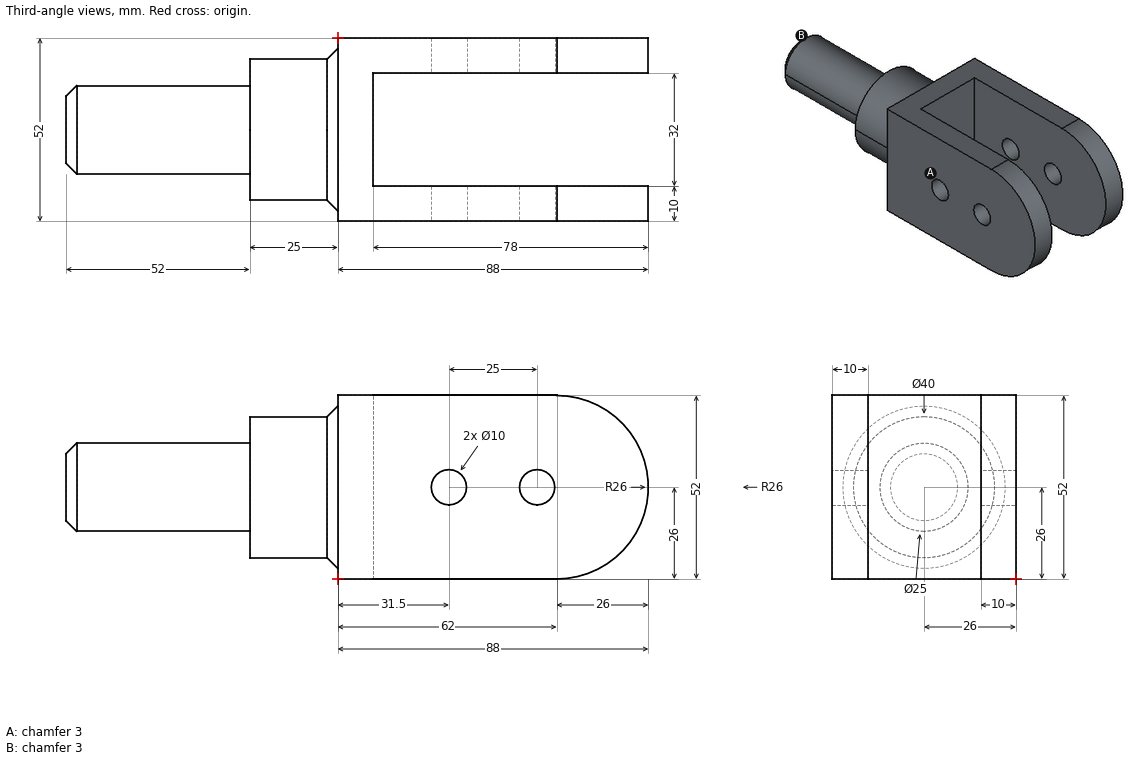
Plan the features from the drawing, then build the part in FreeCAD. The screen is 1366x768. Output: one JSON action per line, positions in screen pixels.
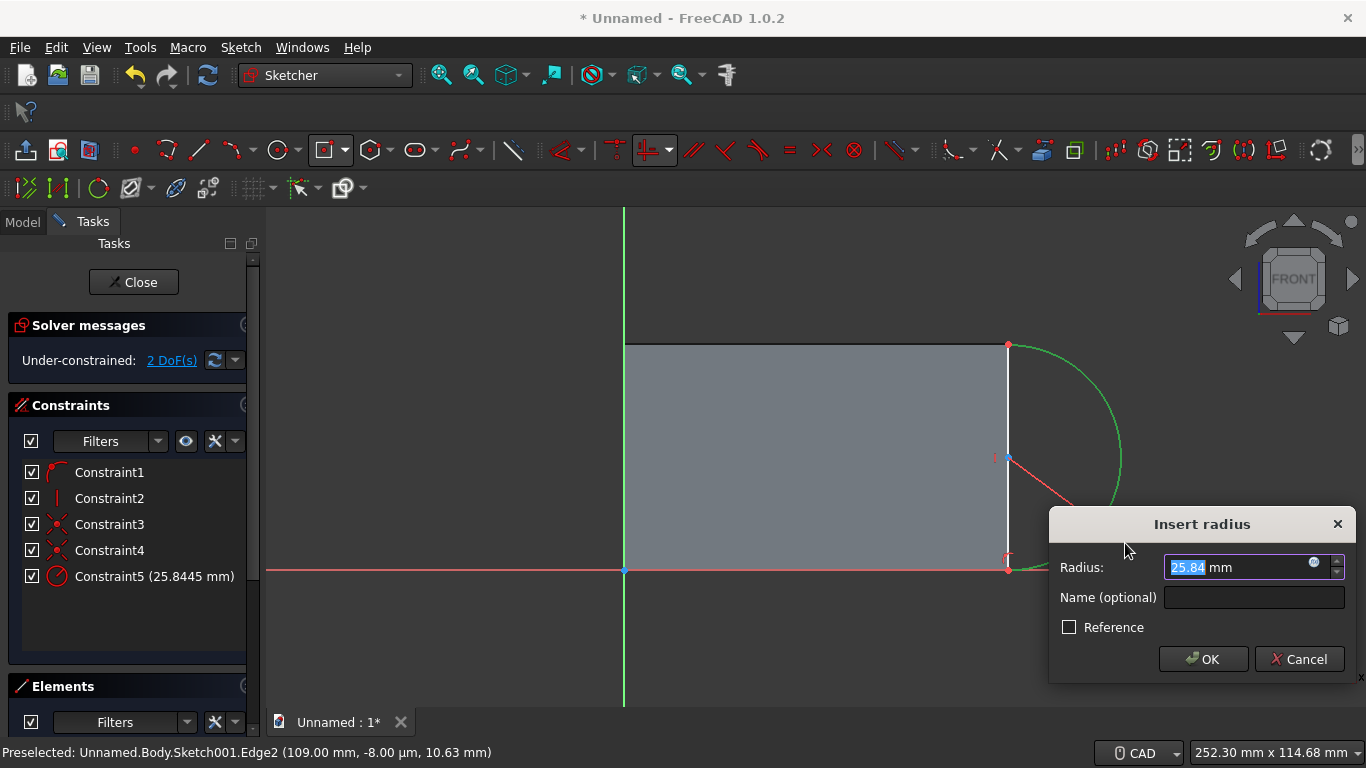
{"action": "type", "text": "26"}
{"action": "key", "text": "Return"}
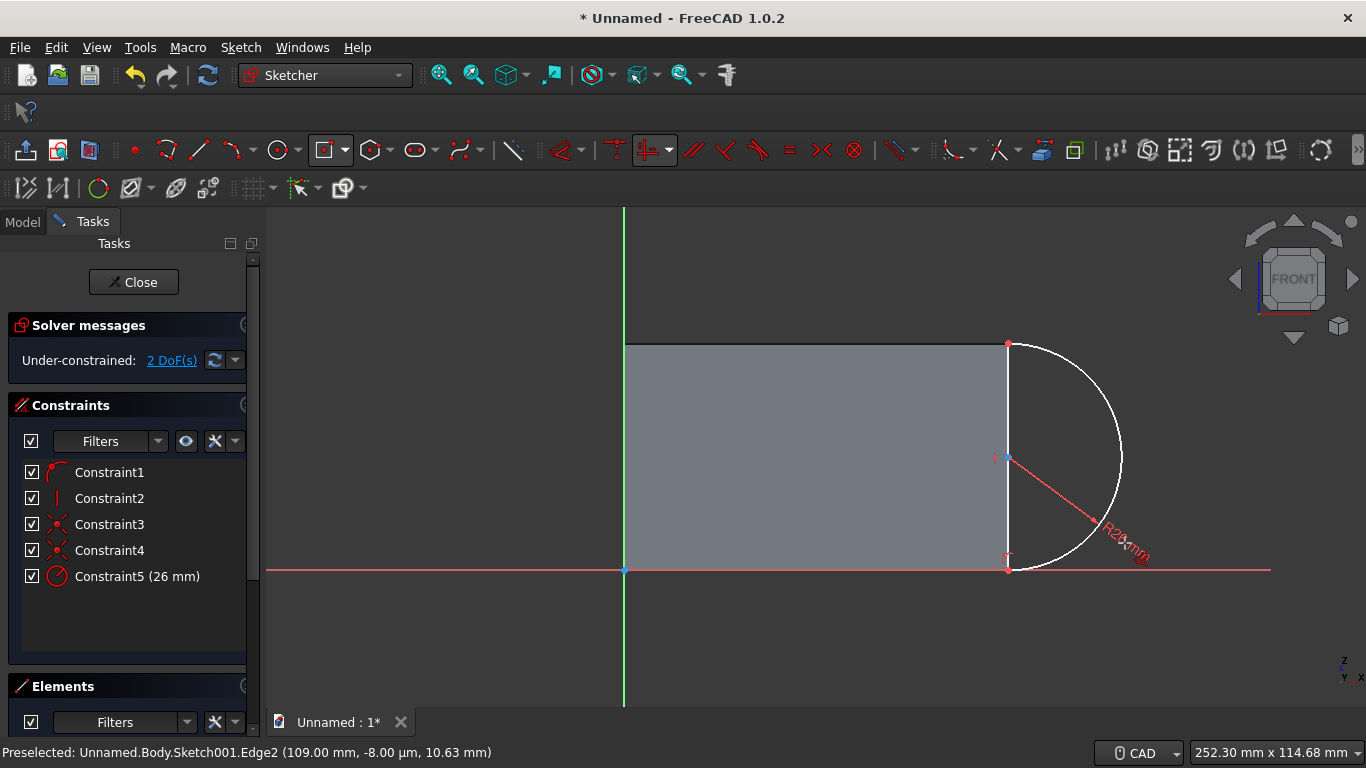
{"action": "left_click", "coordinate": [1008, 570]}
{"action": "left_click", "coordinate": [816, 604]}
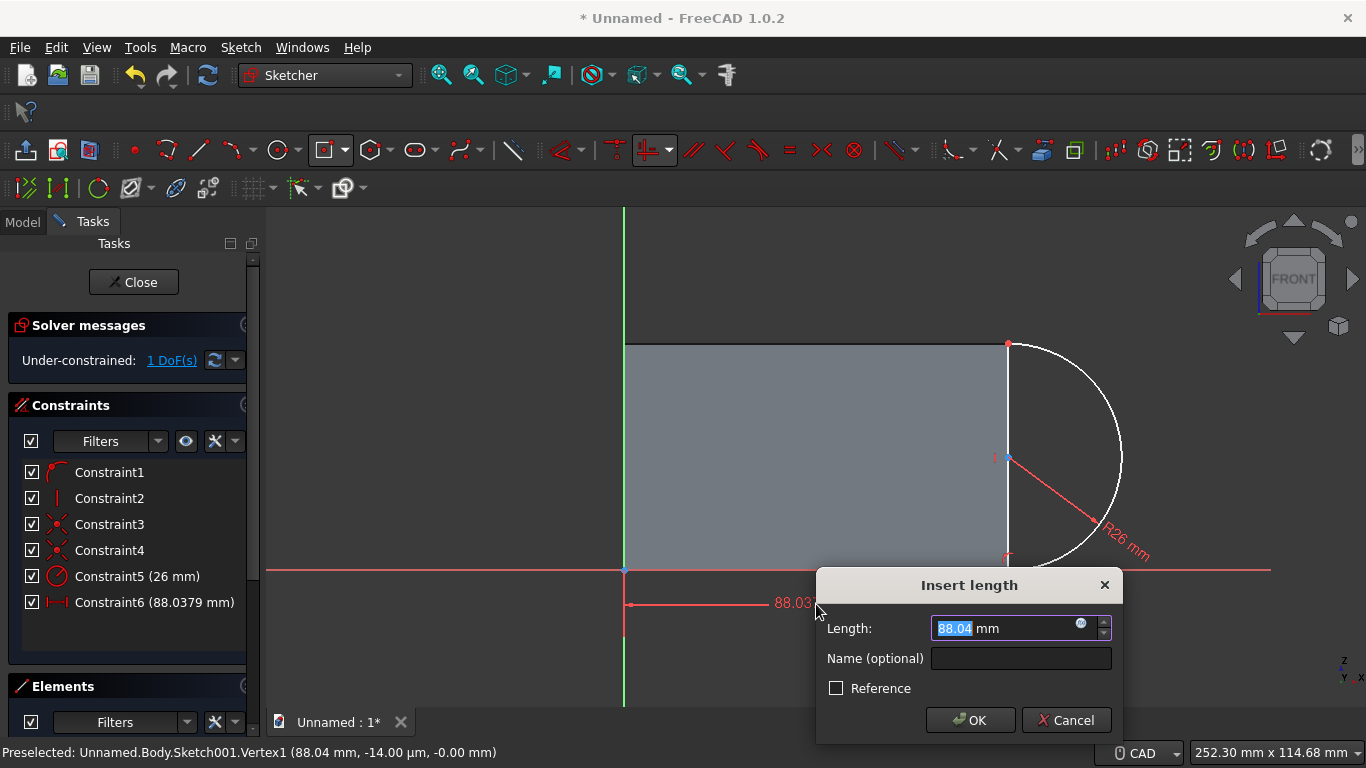
{"action": "type", "text": "88"}
{"action": "key", "text": "Return"}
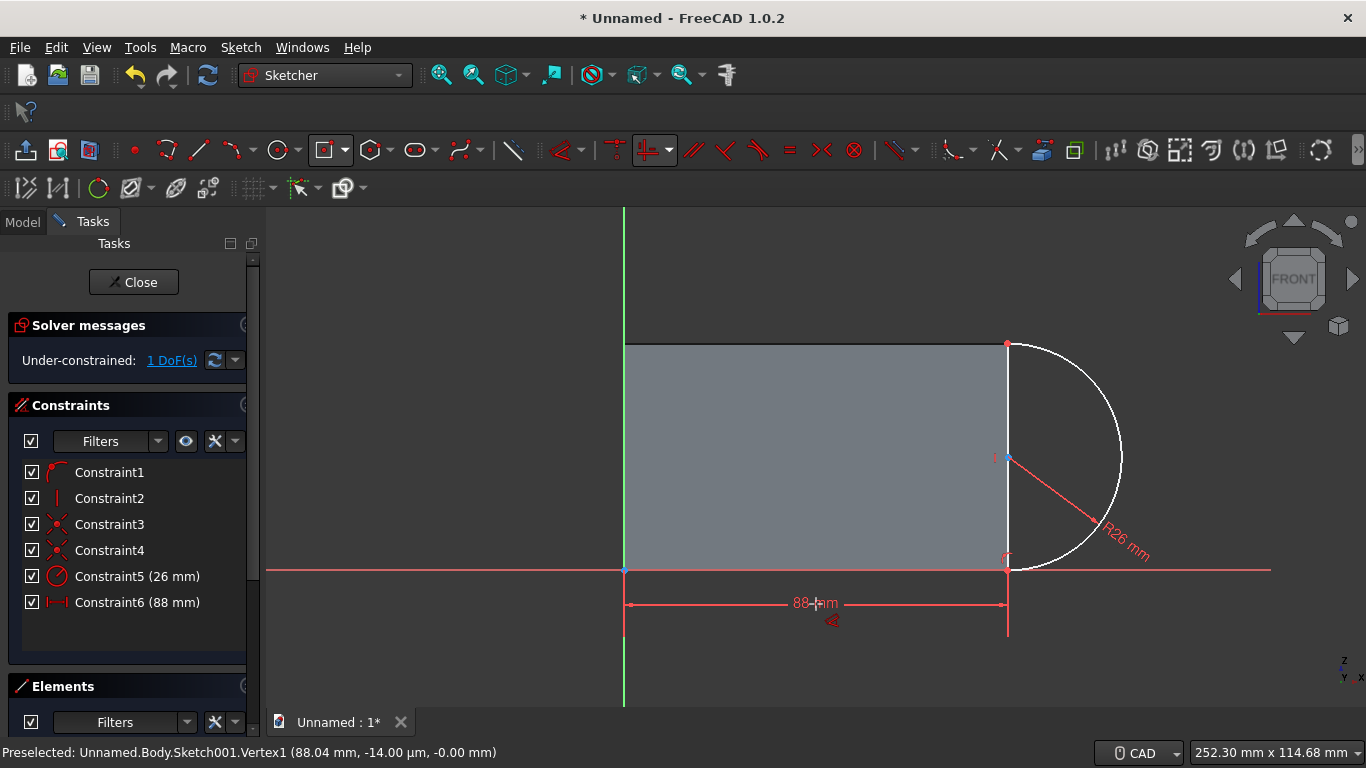
{"action": "left_click", "coordinate": [1008, 457]}
{"action": "left_click", "coordinate": [728, 604]}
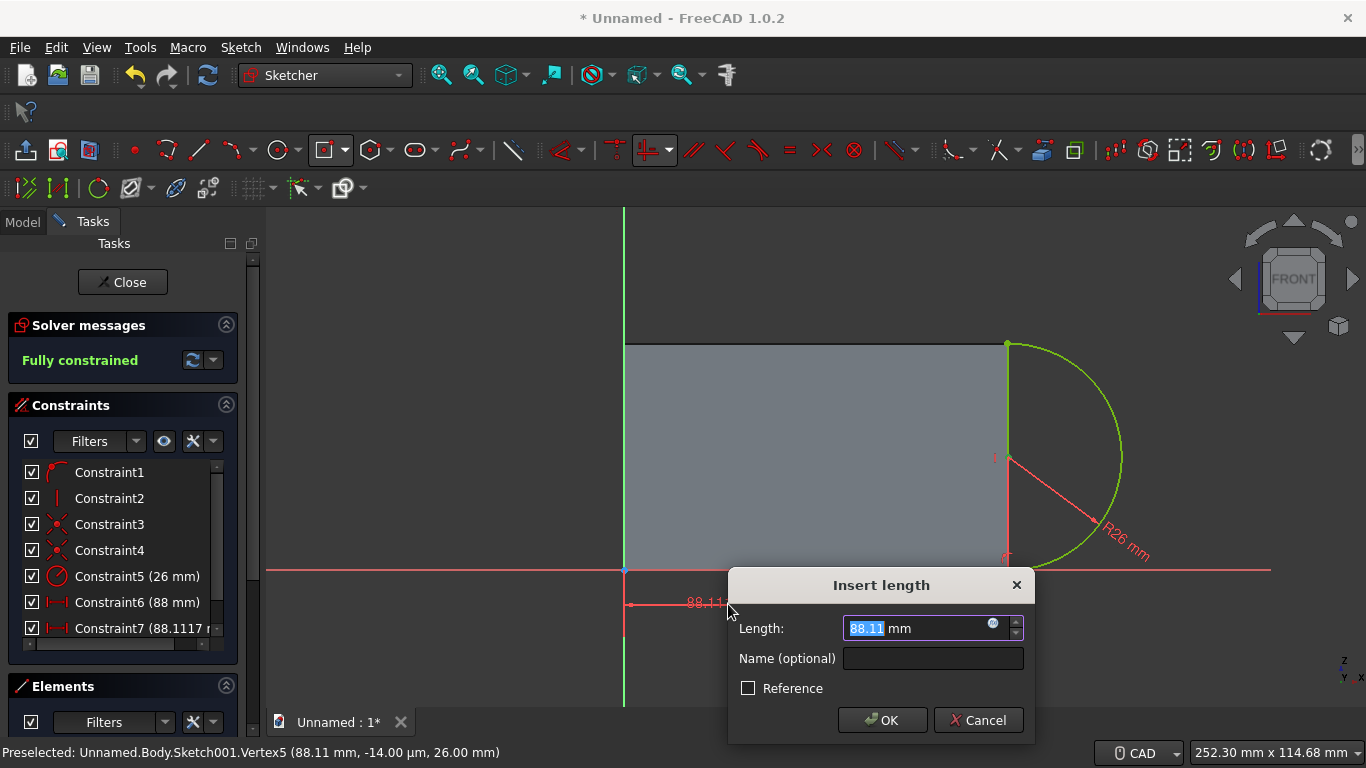
{"action": "type", "text": "88"}
{"action": "key", "text": "Return"}
{"action": "key", "text": "Escape"}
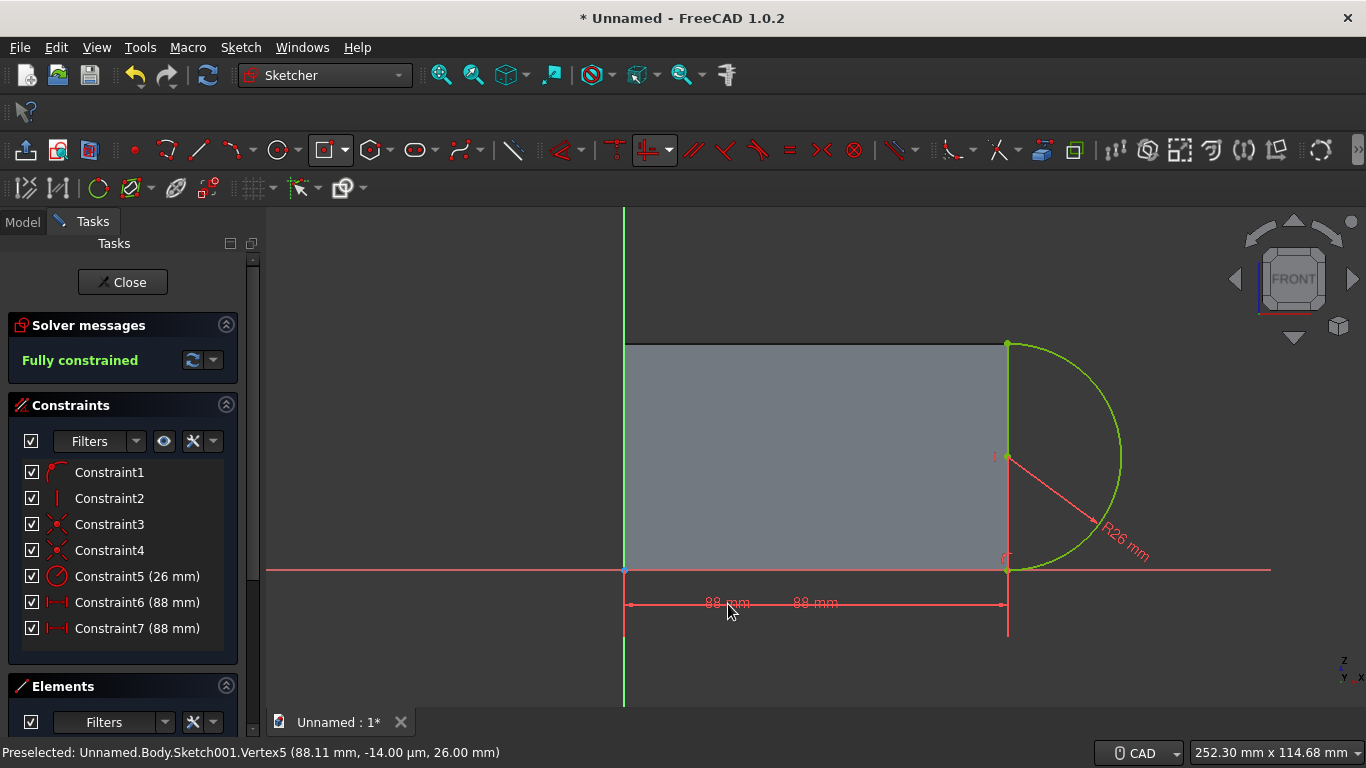
{"action": "left_click", "coordinate": [123, 282]}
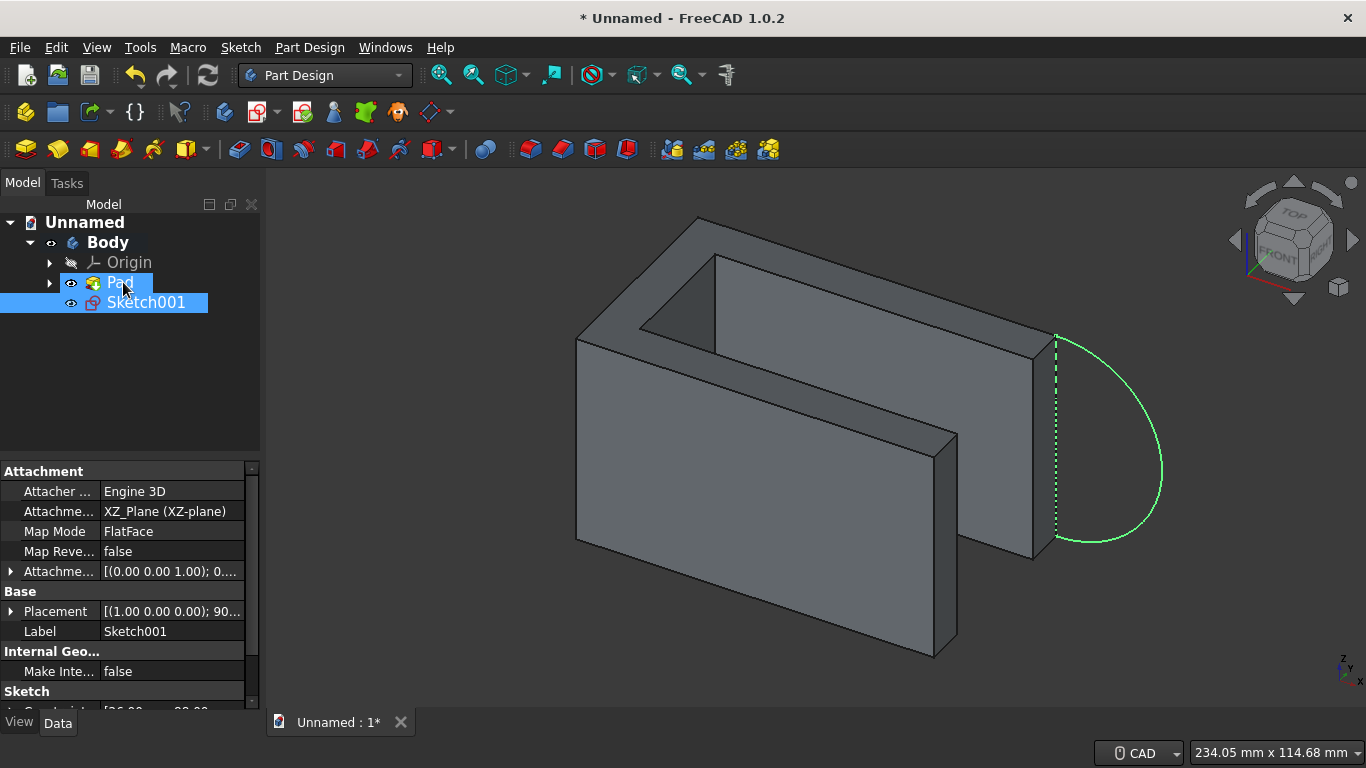
{"action": "left_click", "coordinate": [26, 150]}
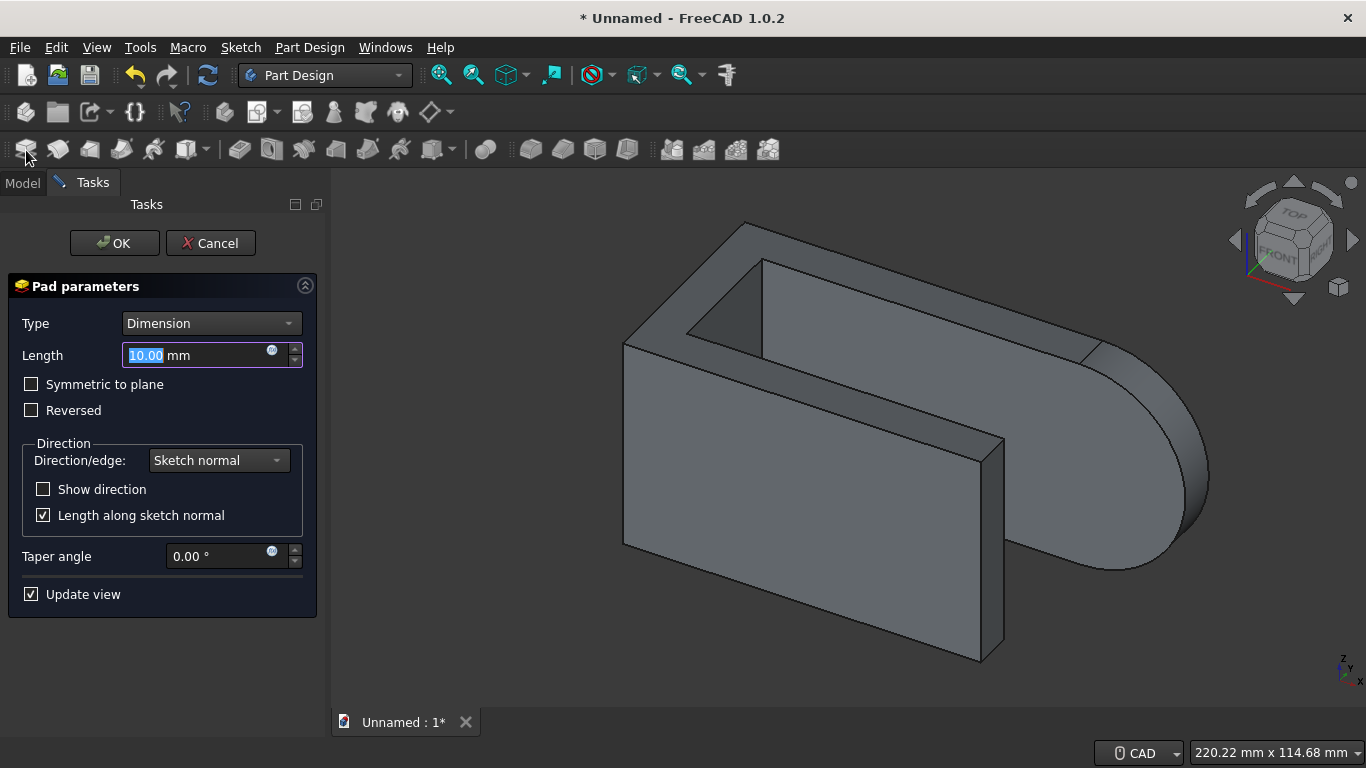
{"action": "type", "text": "10"}
{"action": "key", "text": "Tab"}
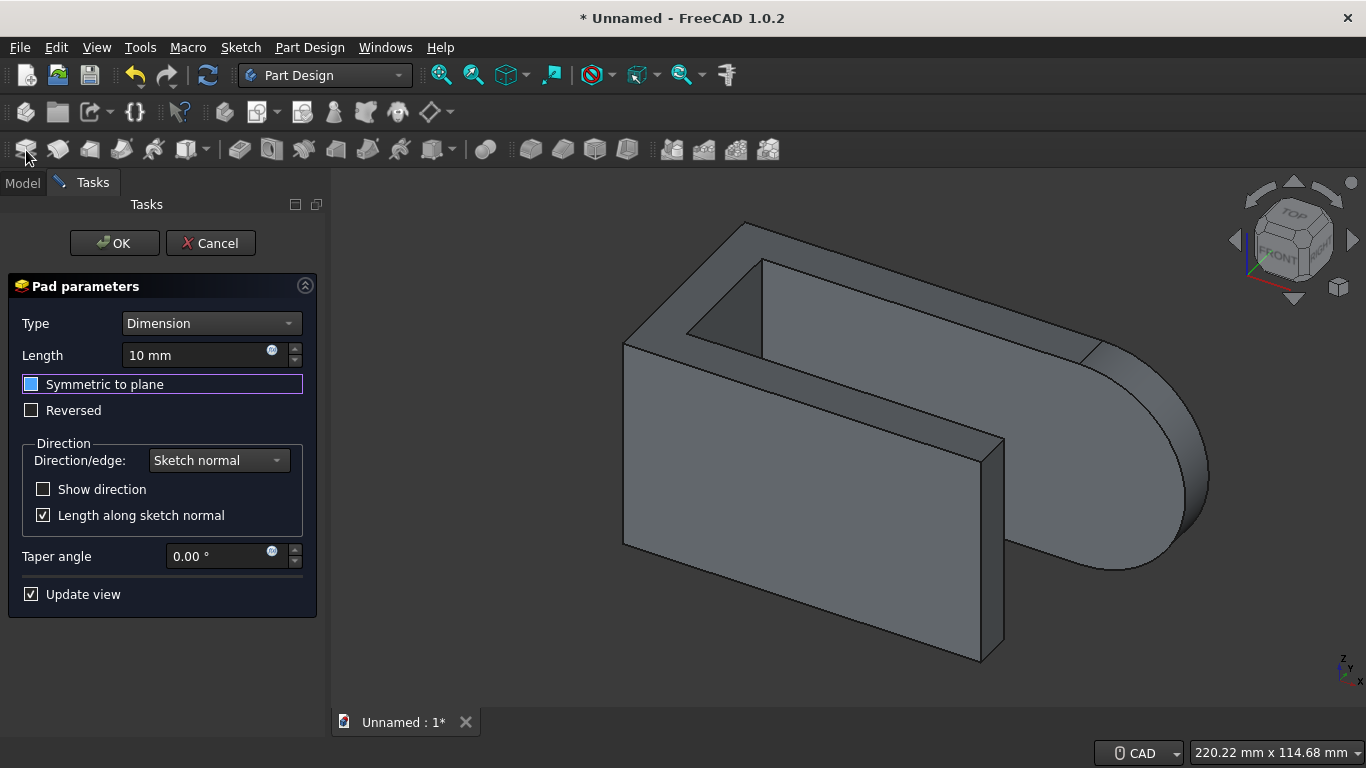
{"action": "left_click", "coordinate": [115, 243]}